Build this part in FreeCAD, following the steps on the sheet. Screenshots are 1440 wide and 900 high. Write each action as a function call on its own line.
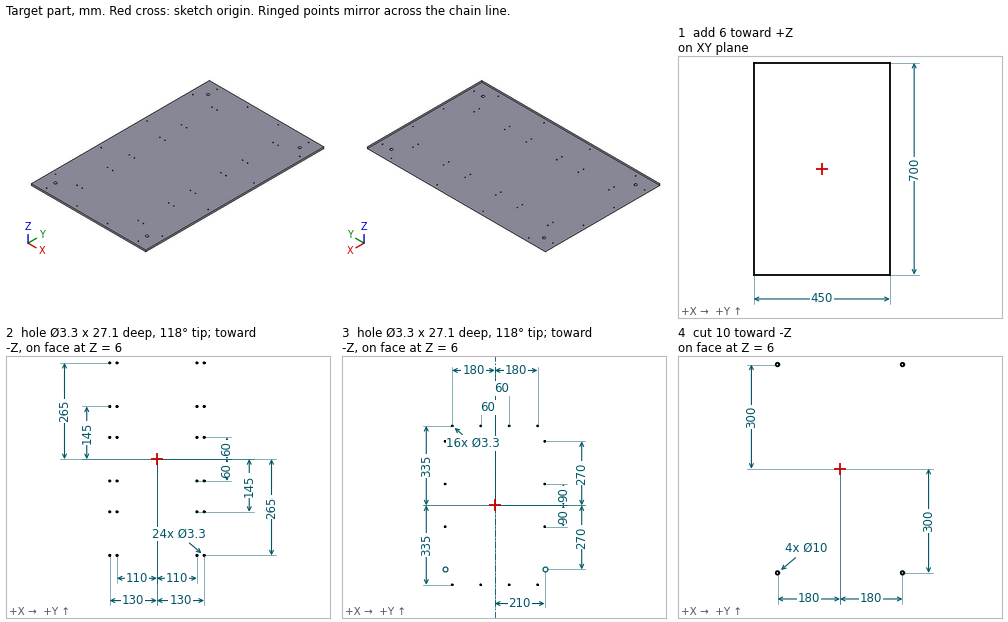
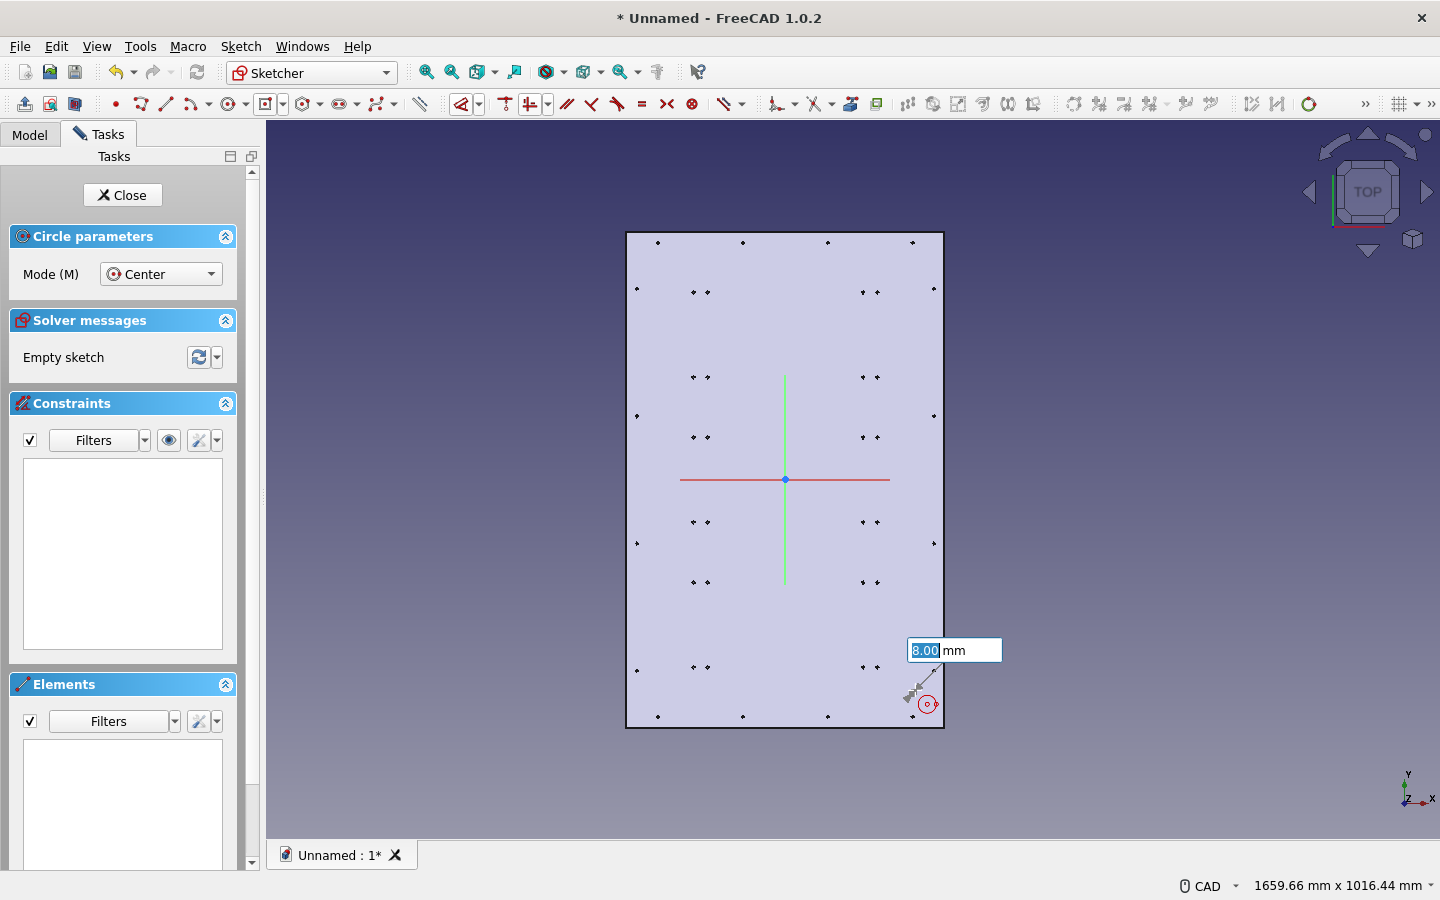
text(10)
key(Return)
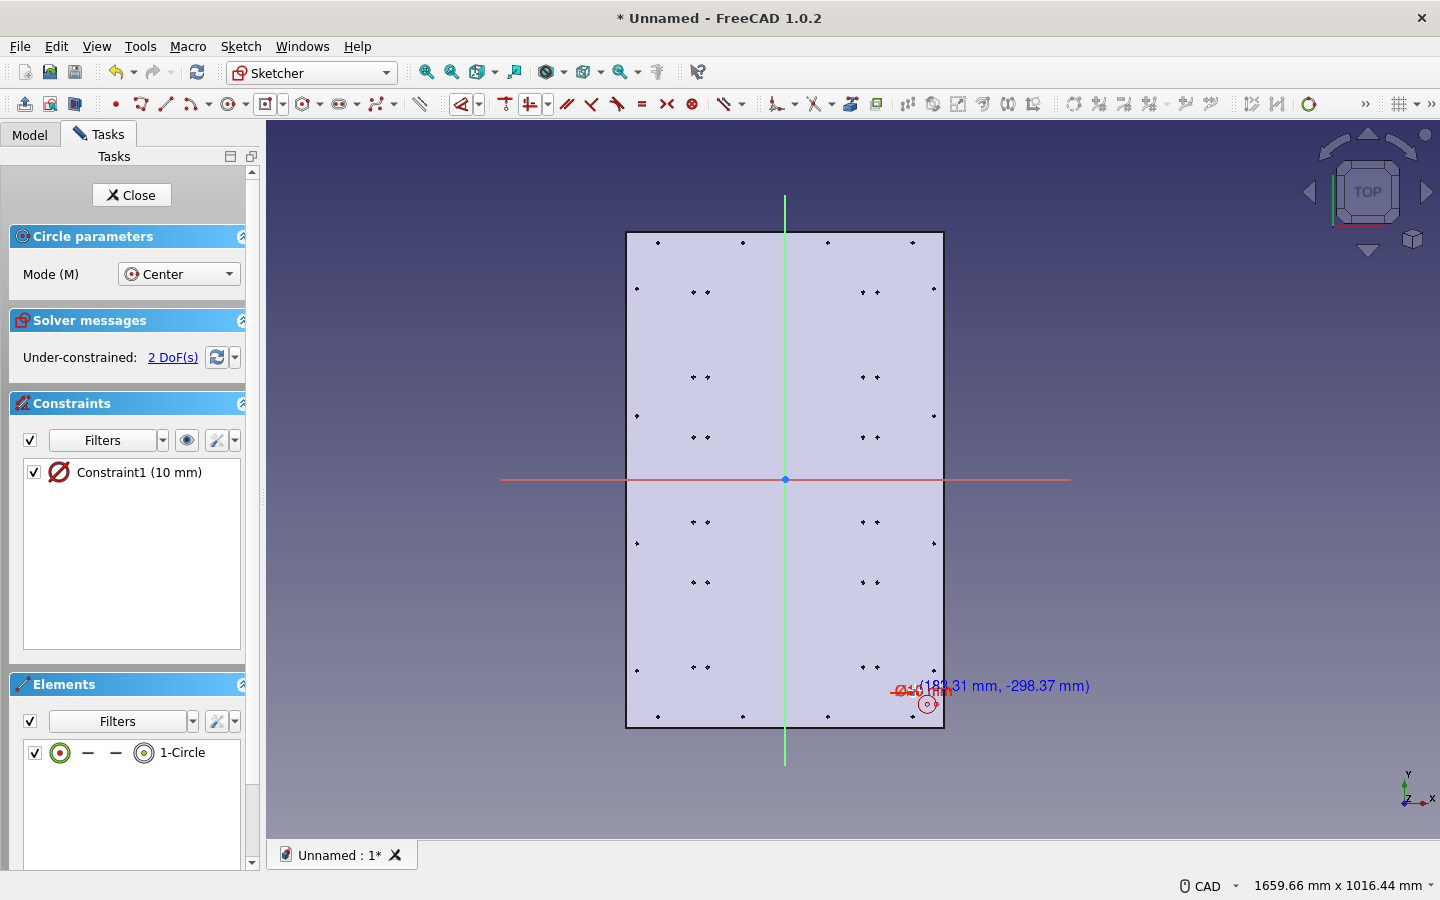
scroll(658, 692, up, 10)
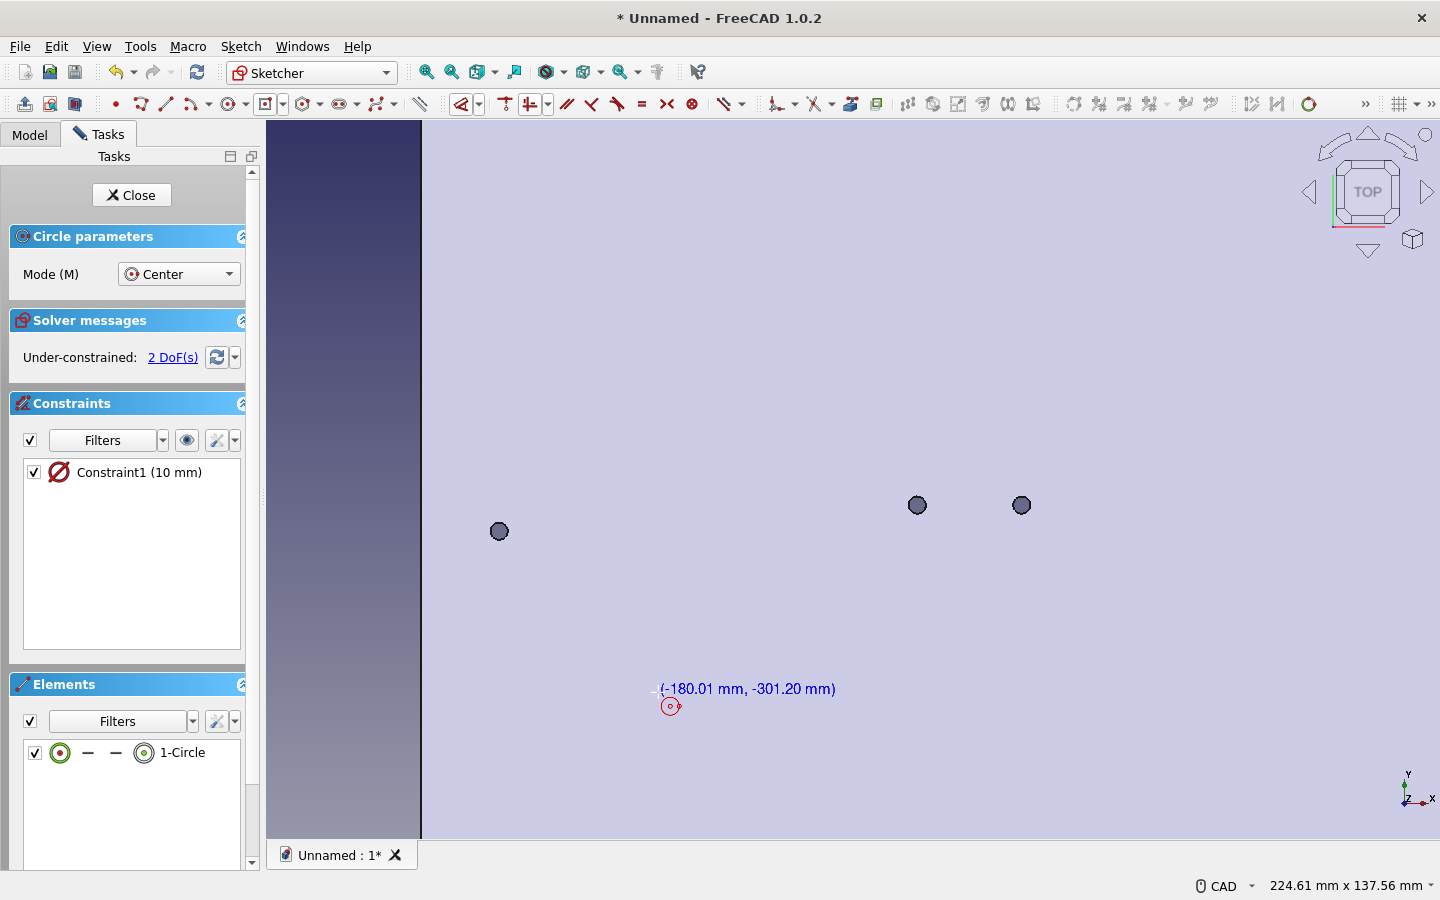
scroll(657, 692, down, 10)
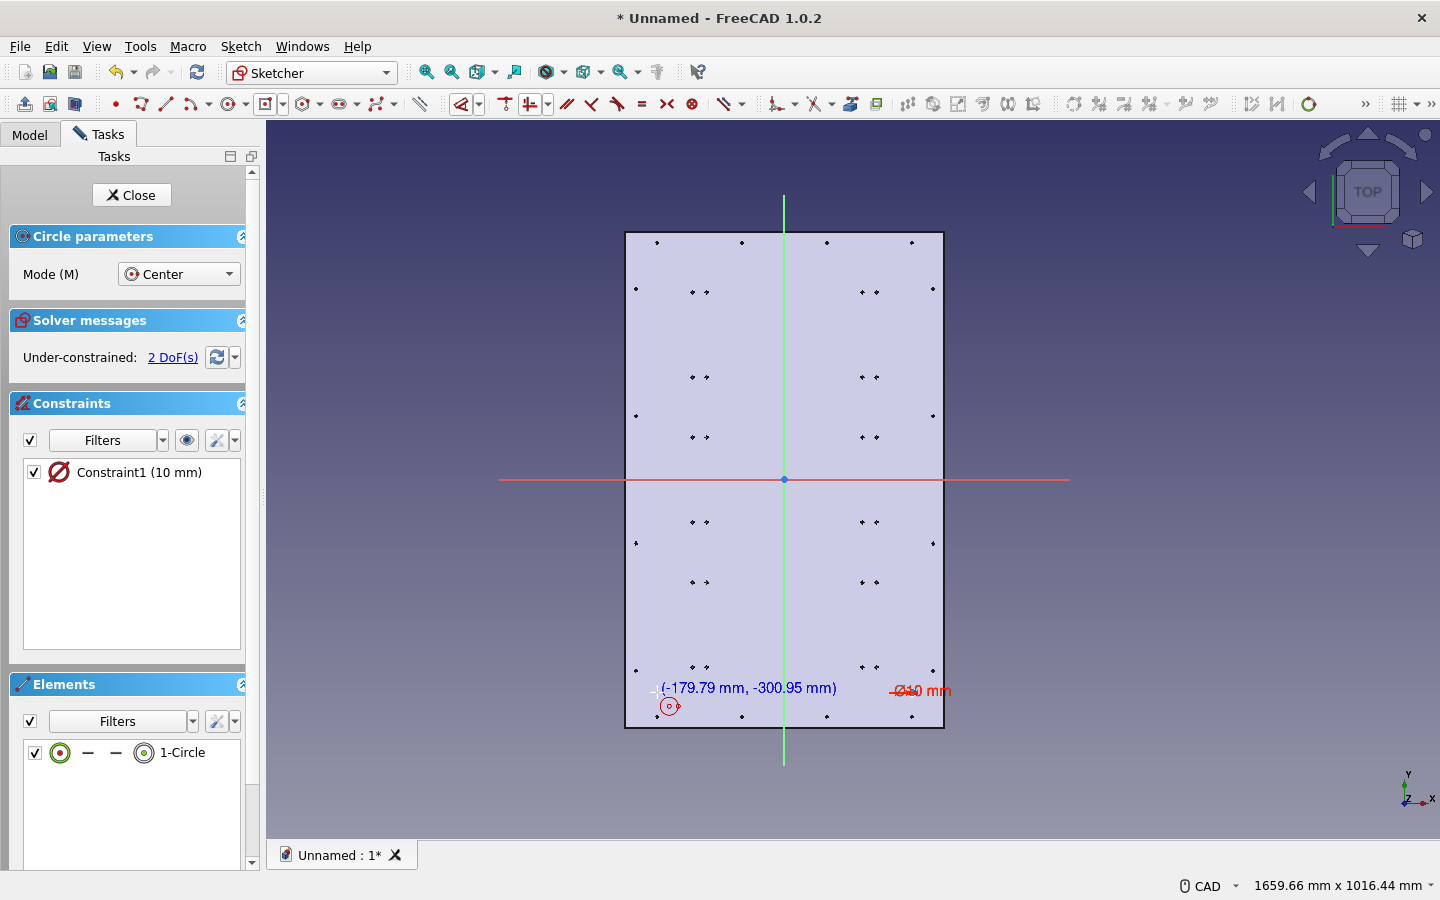
click(657, 692)
move(660, 690)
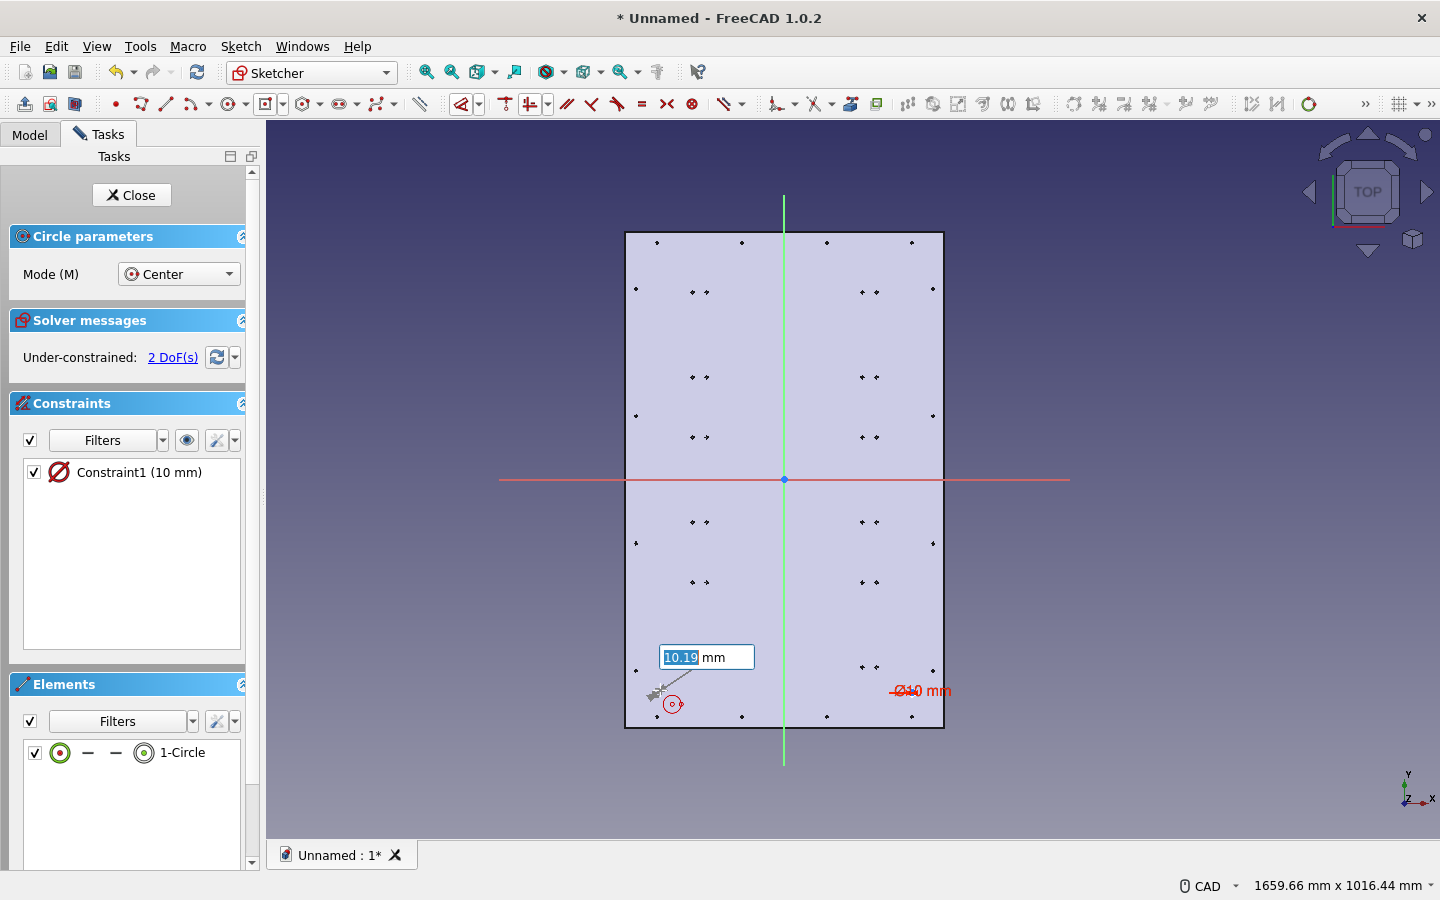
text(10)
key(Return)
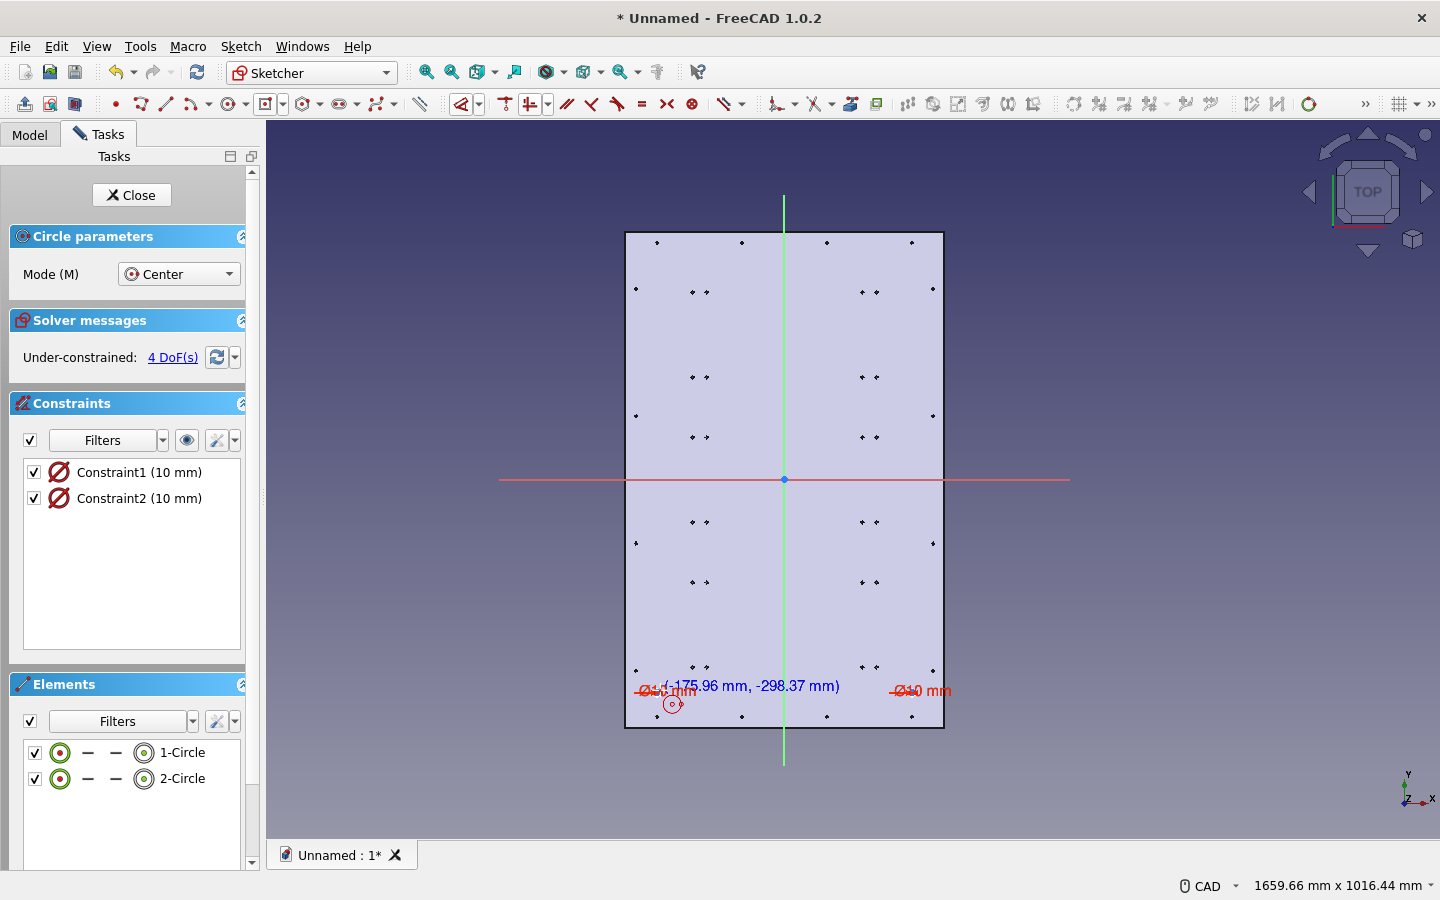
scroll(657, 268, up, 10)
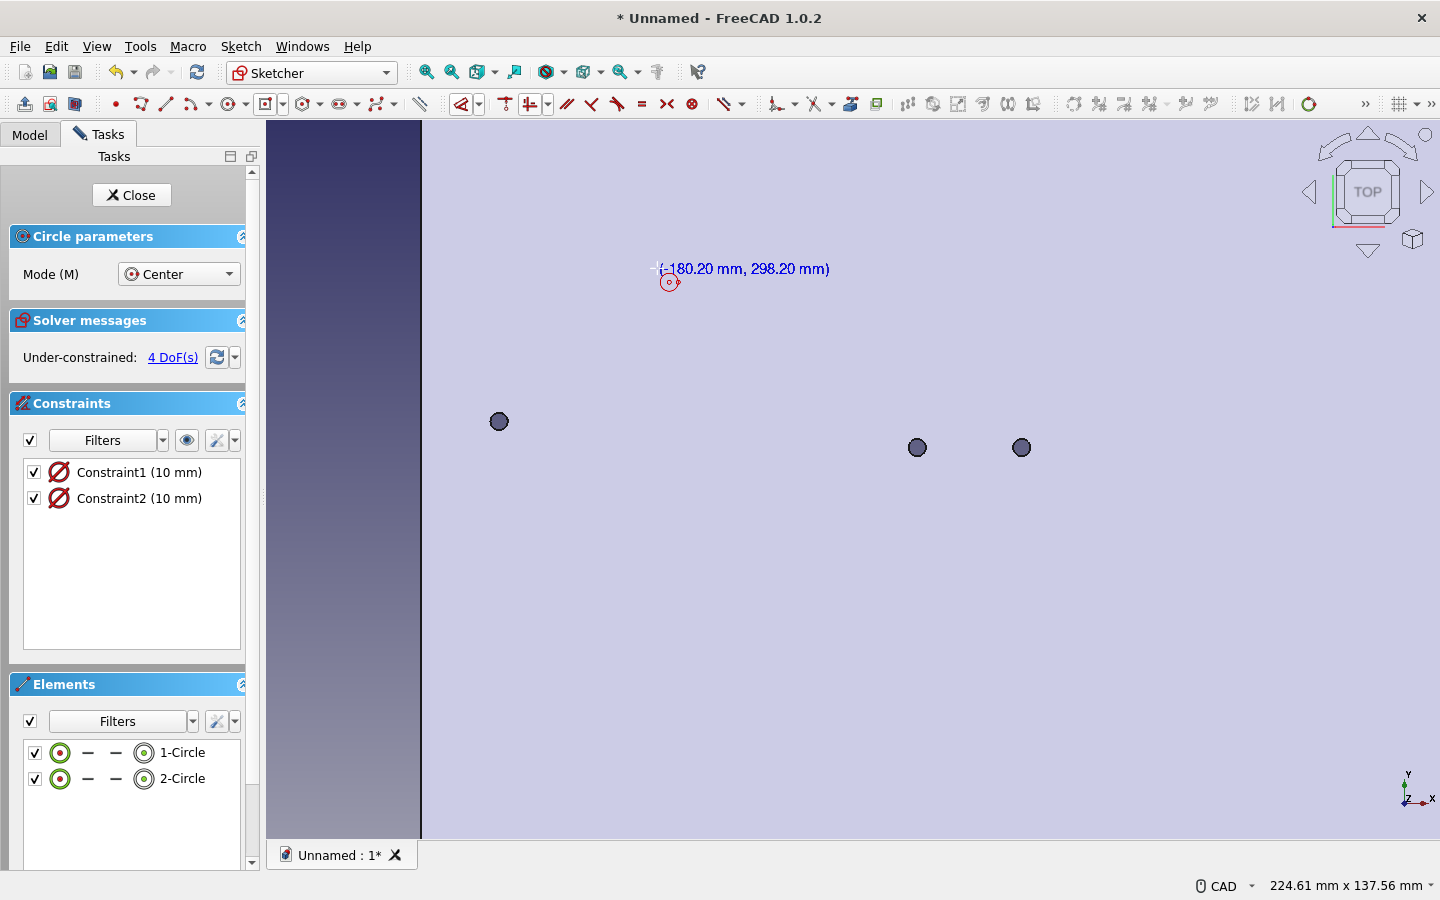
scroll(657, 268, down, 10)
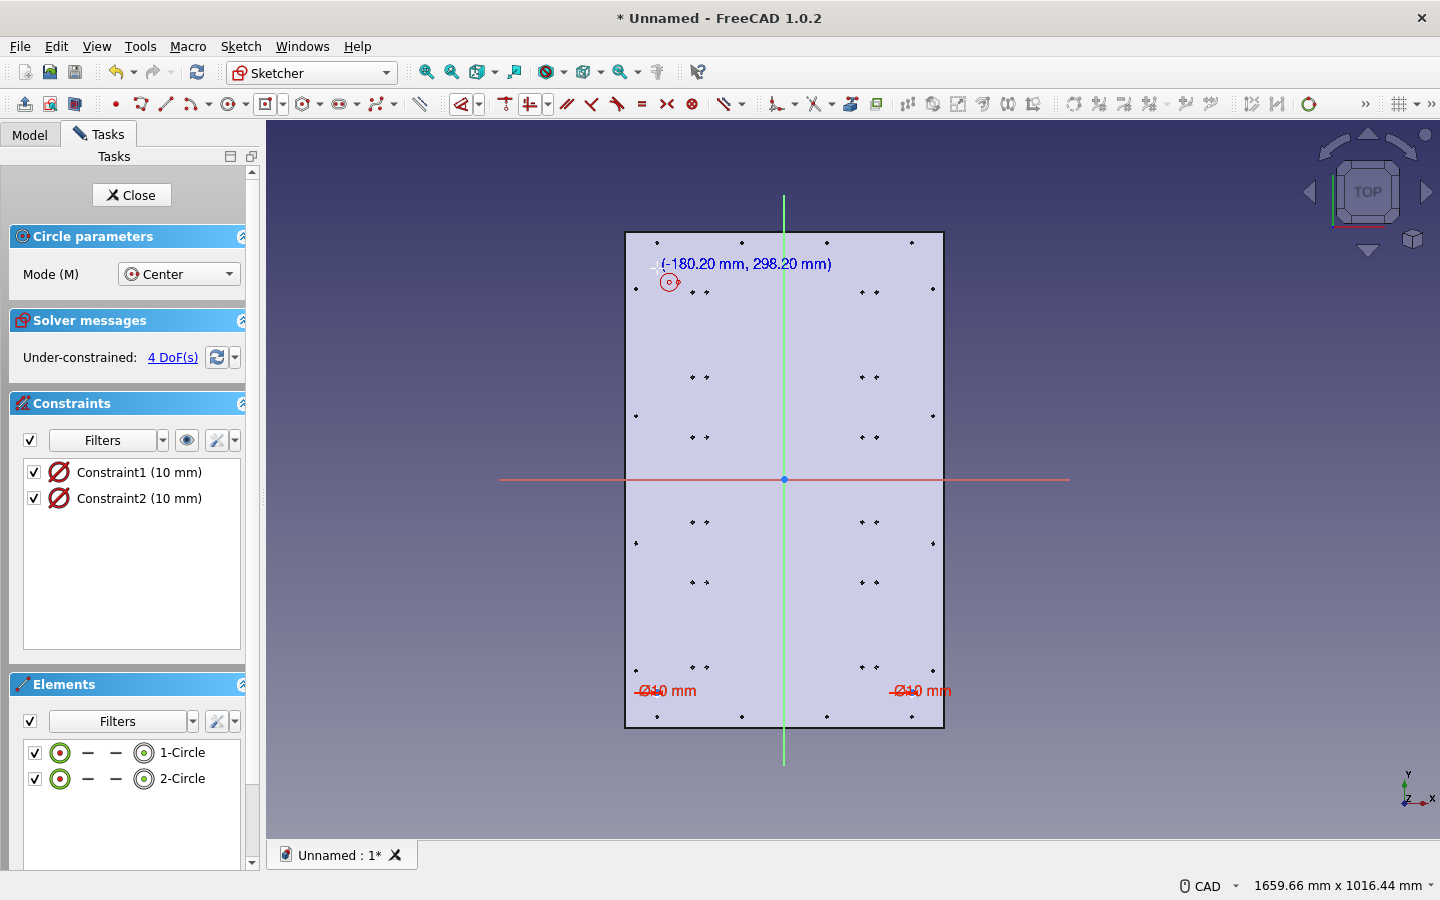
click(657, 268)
move(660, 265)